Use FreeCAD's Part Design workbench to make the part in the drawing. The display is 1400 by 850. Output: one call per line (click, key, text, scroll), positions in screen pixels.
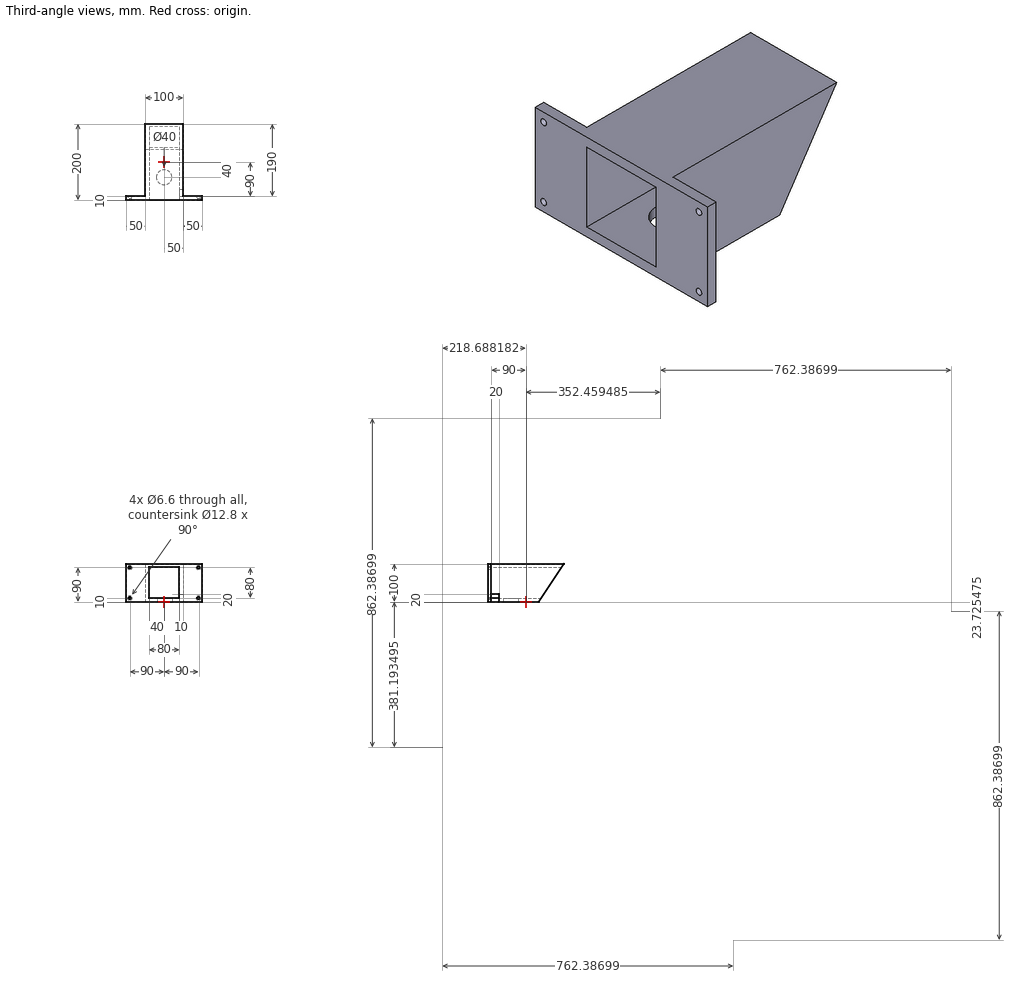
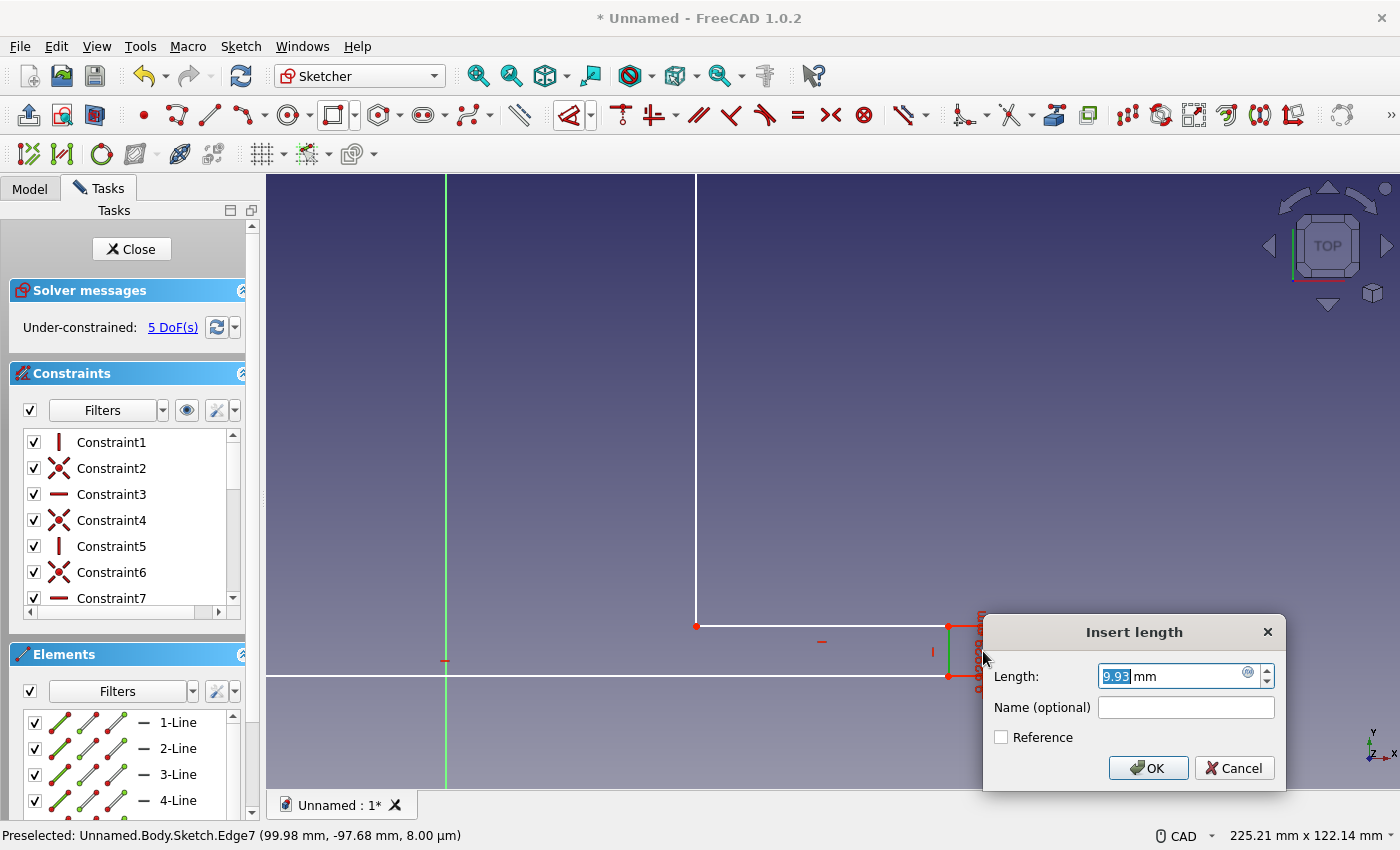
text(10)
key(Return)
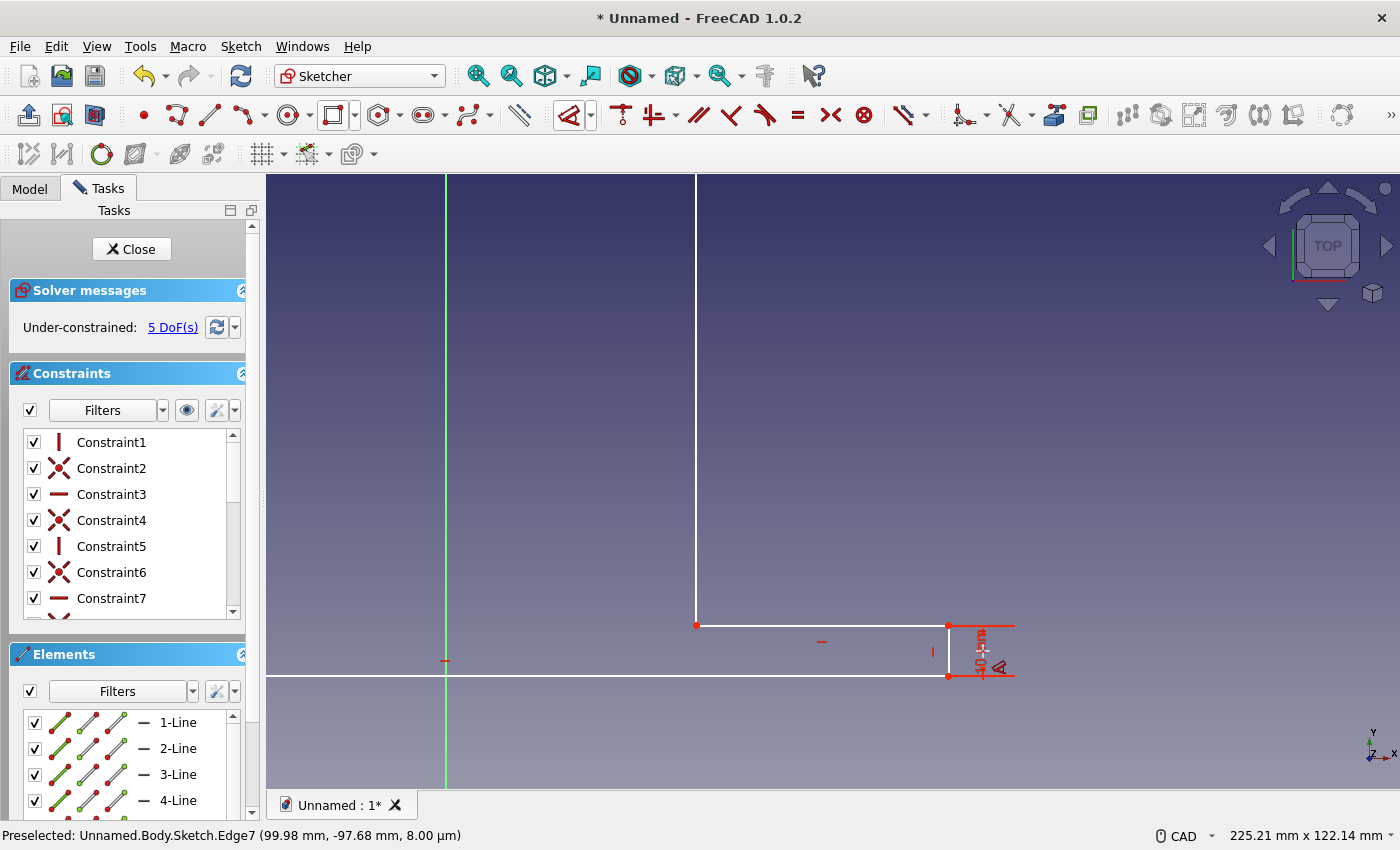
click(873, 626)
click(823, 660)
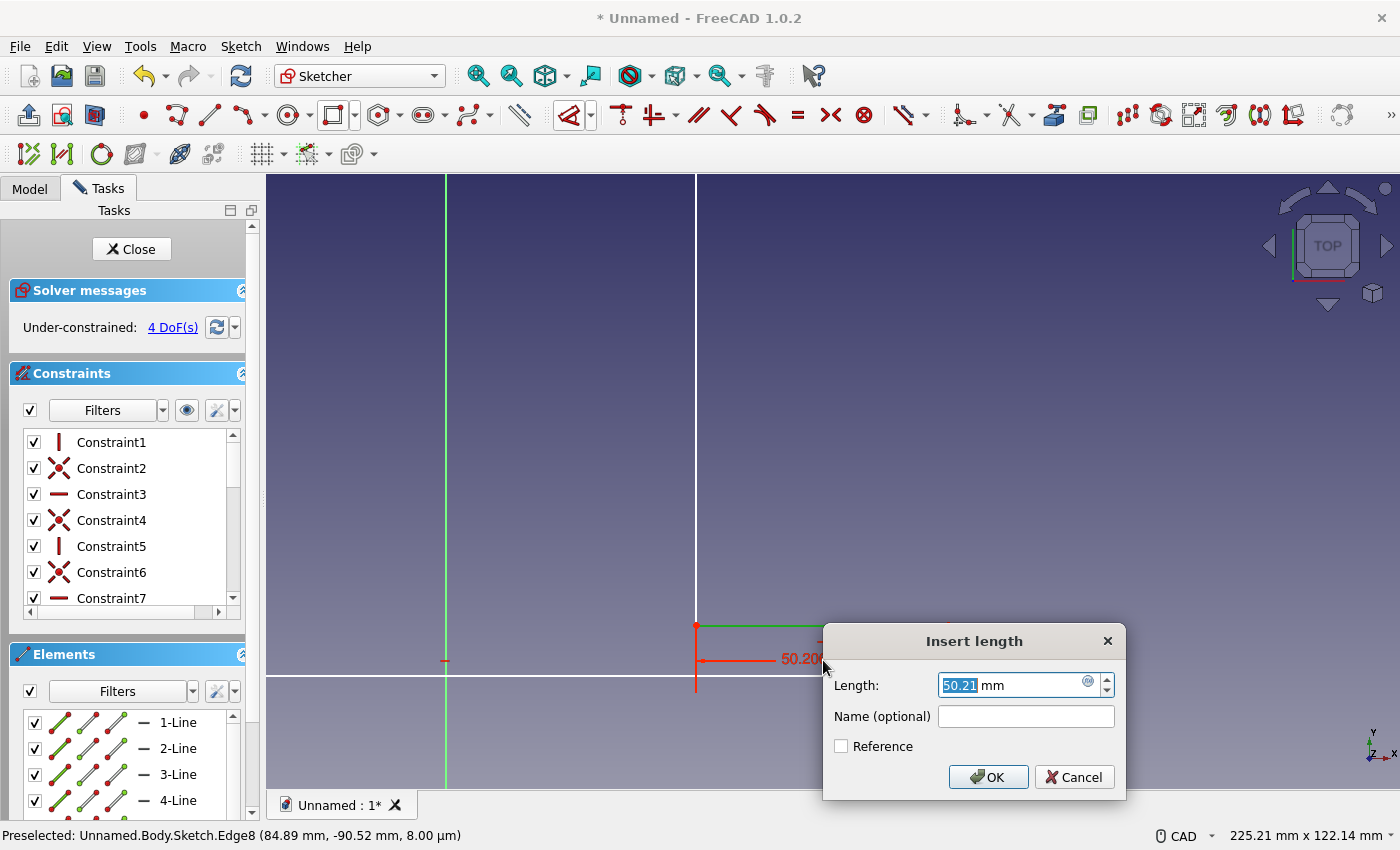
text(50)
key(Return)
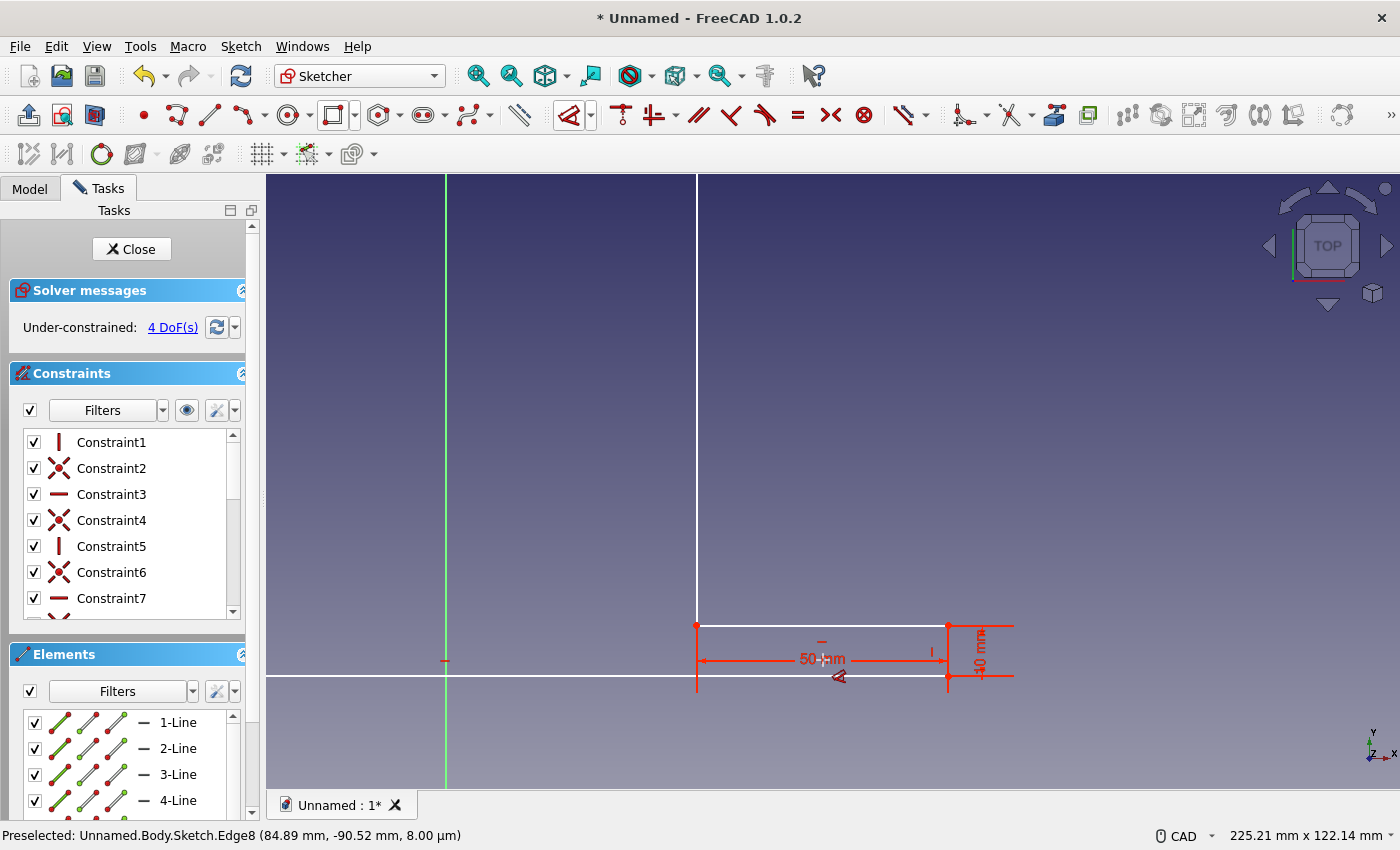
click(697, 339)
click(731, 414)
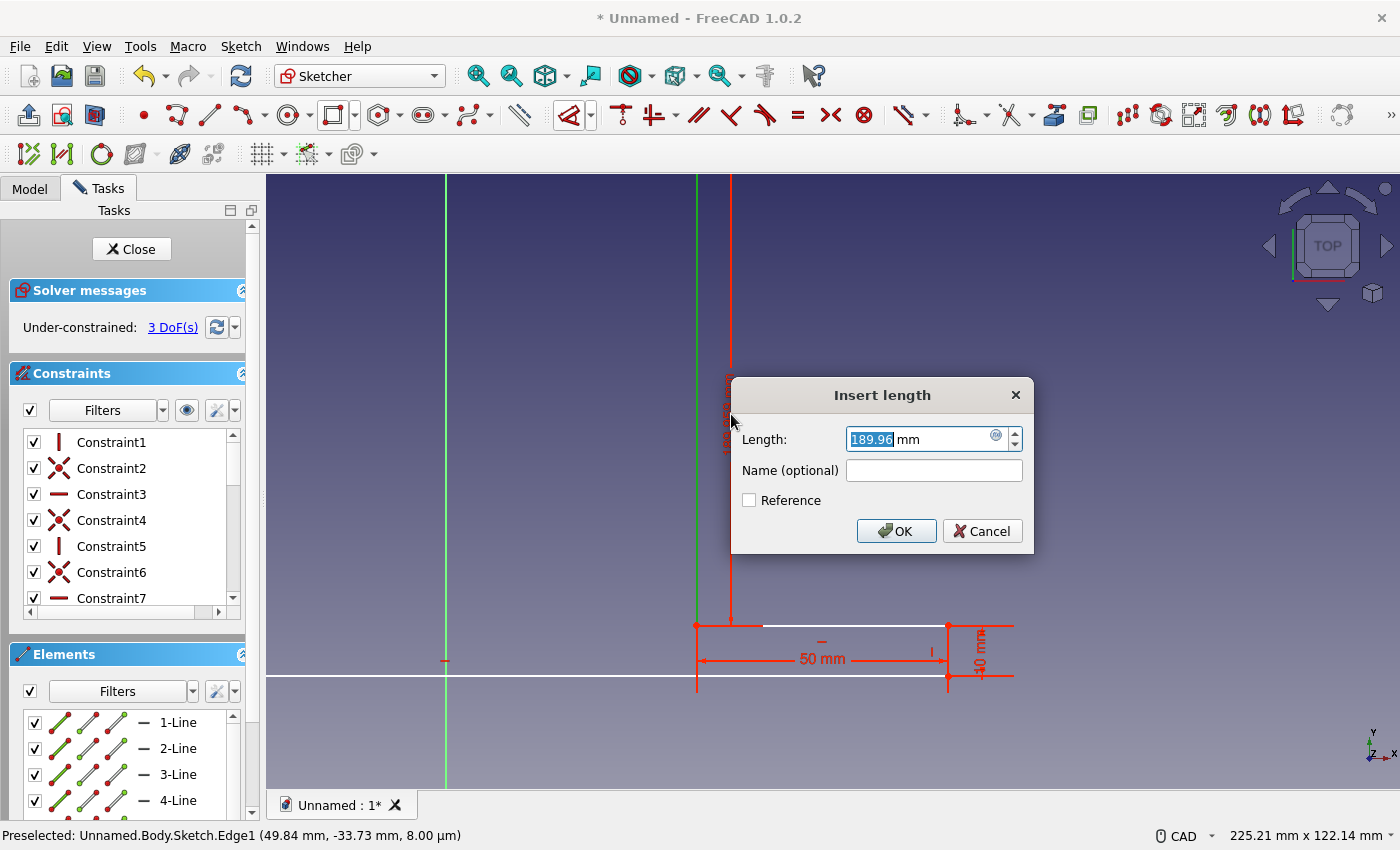
text(190)
key(Return)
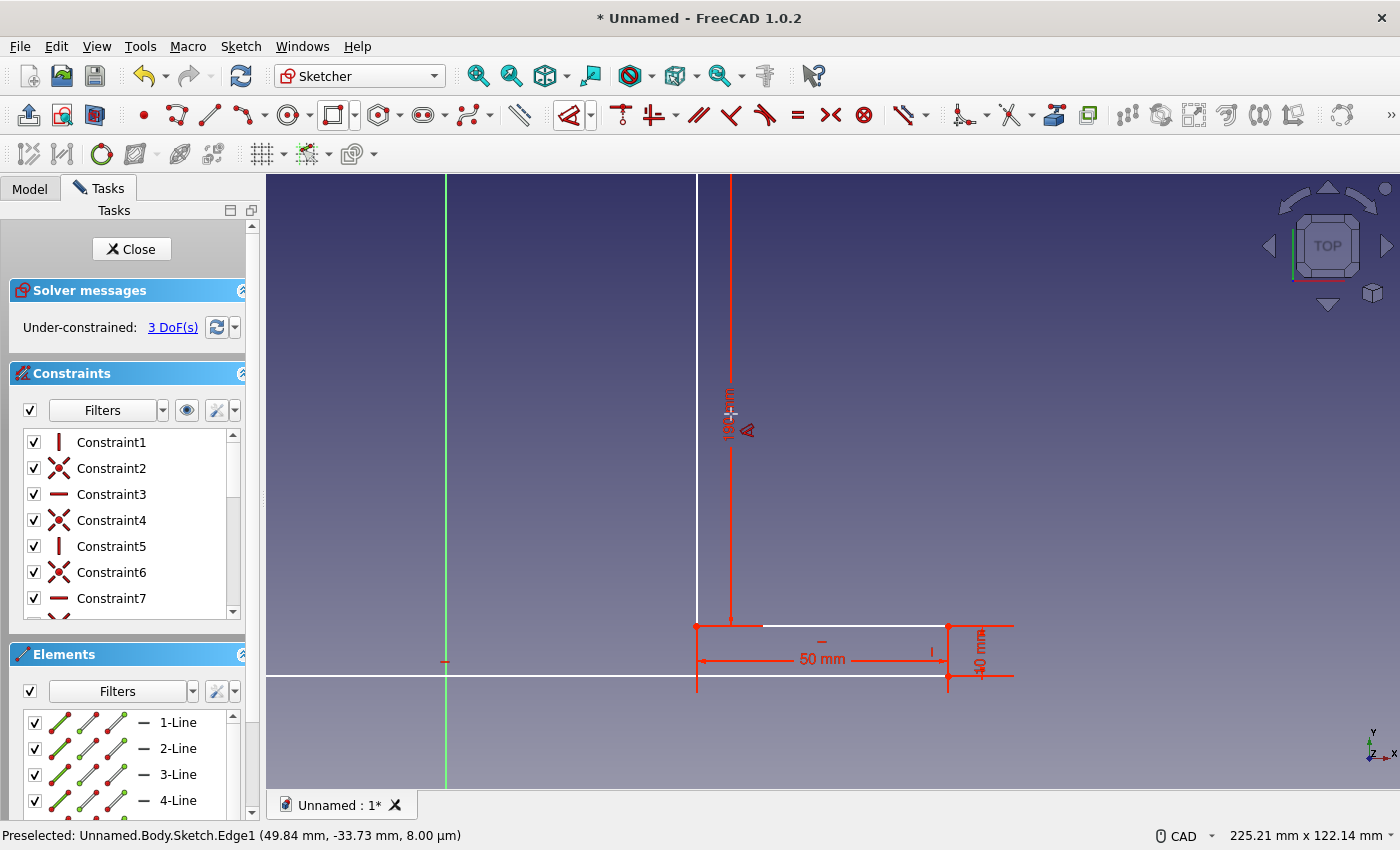
scroll(950, 663, down, 5)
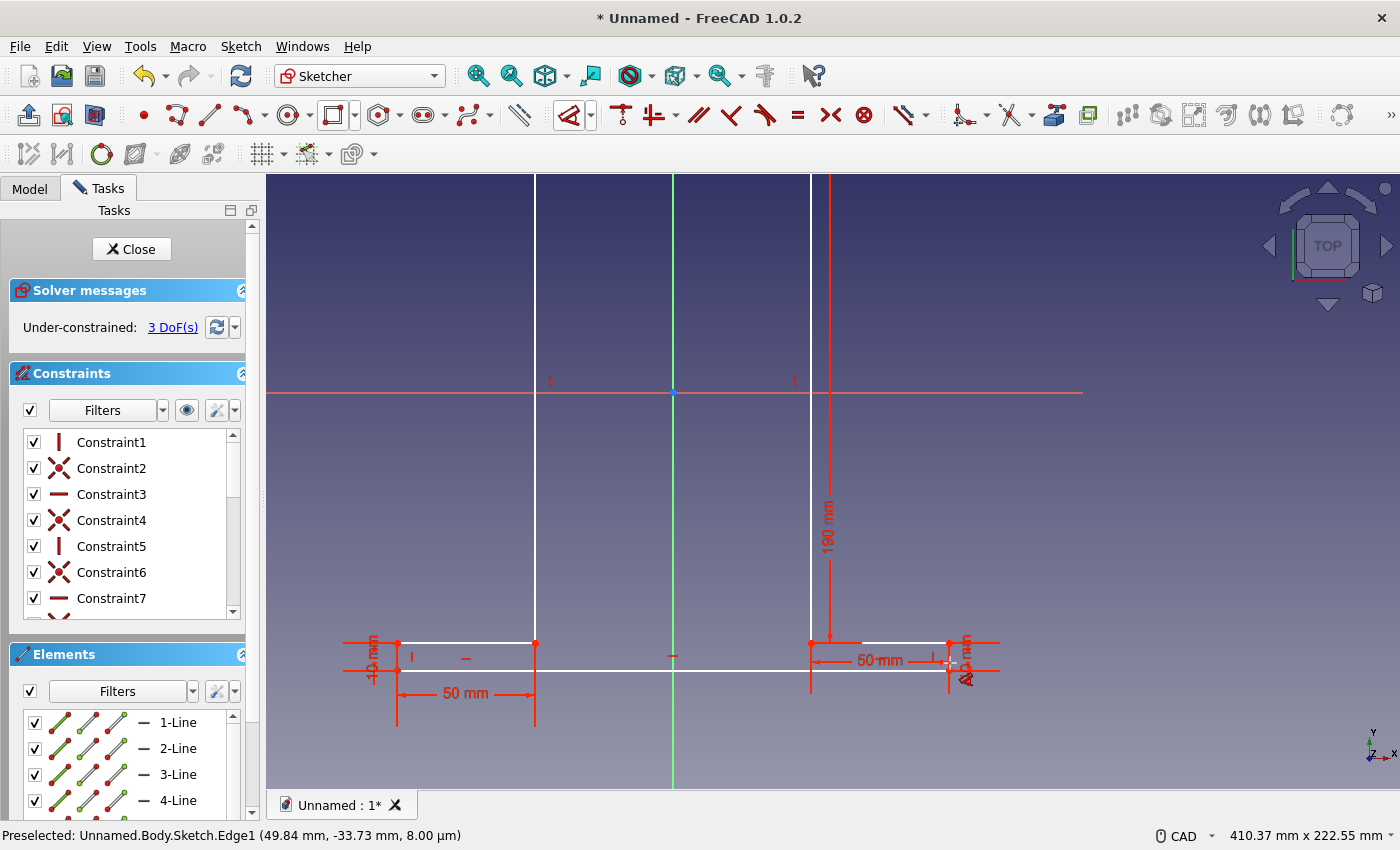
click(802, 298)
click(722, 264)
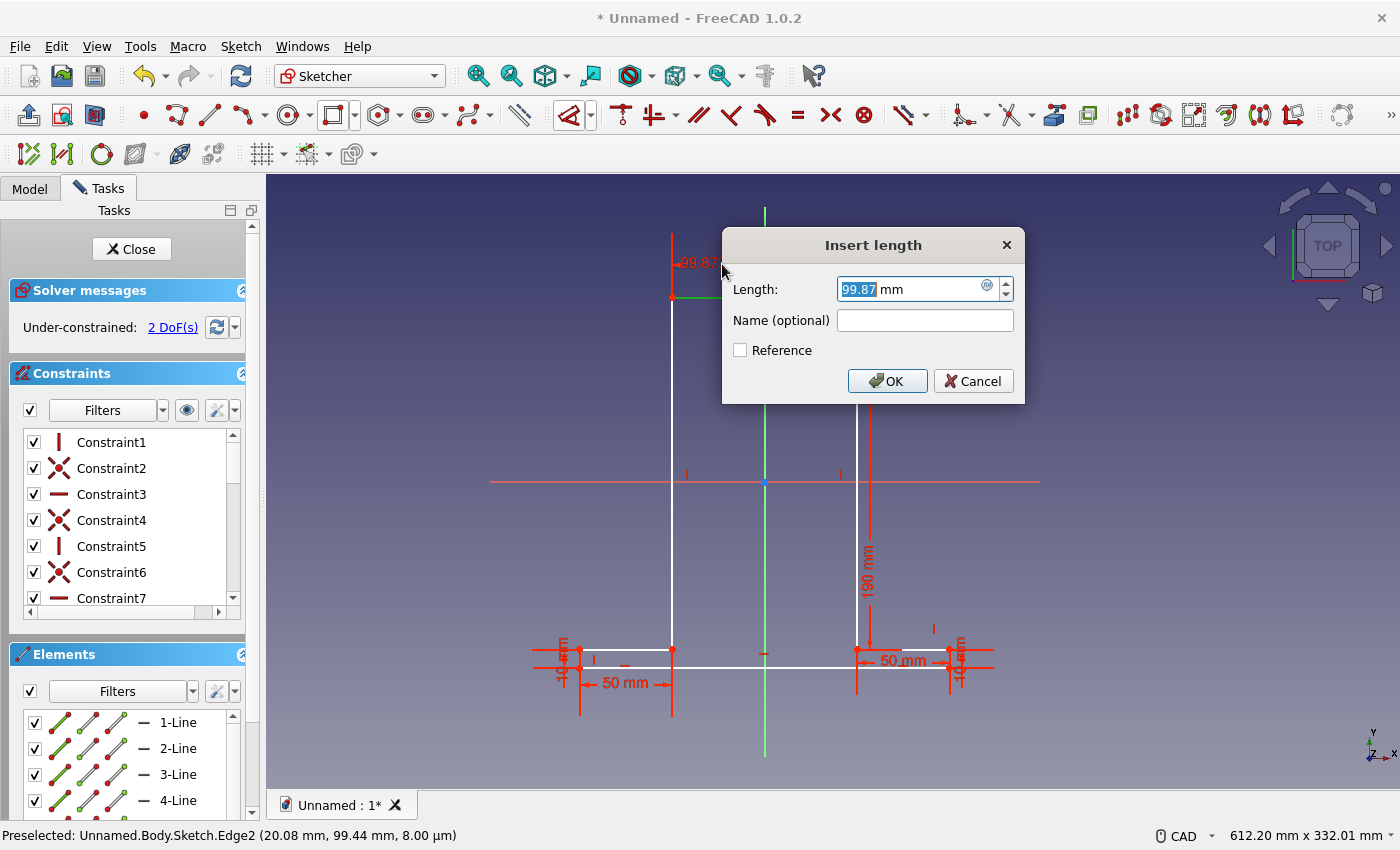
text(100)
key(Return)